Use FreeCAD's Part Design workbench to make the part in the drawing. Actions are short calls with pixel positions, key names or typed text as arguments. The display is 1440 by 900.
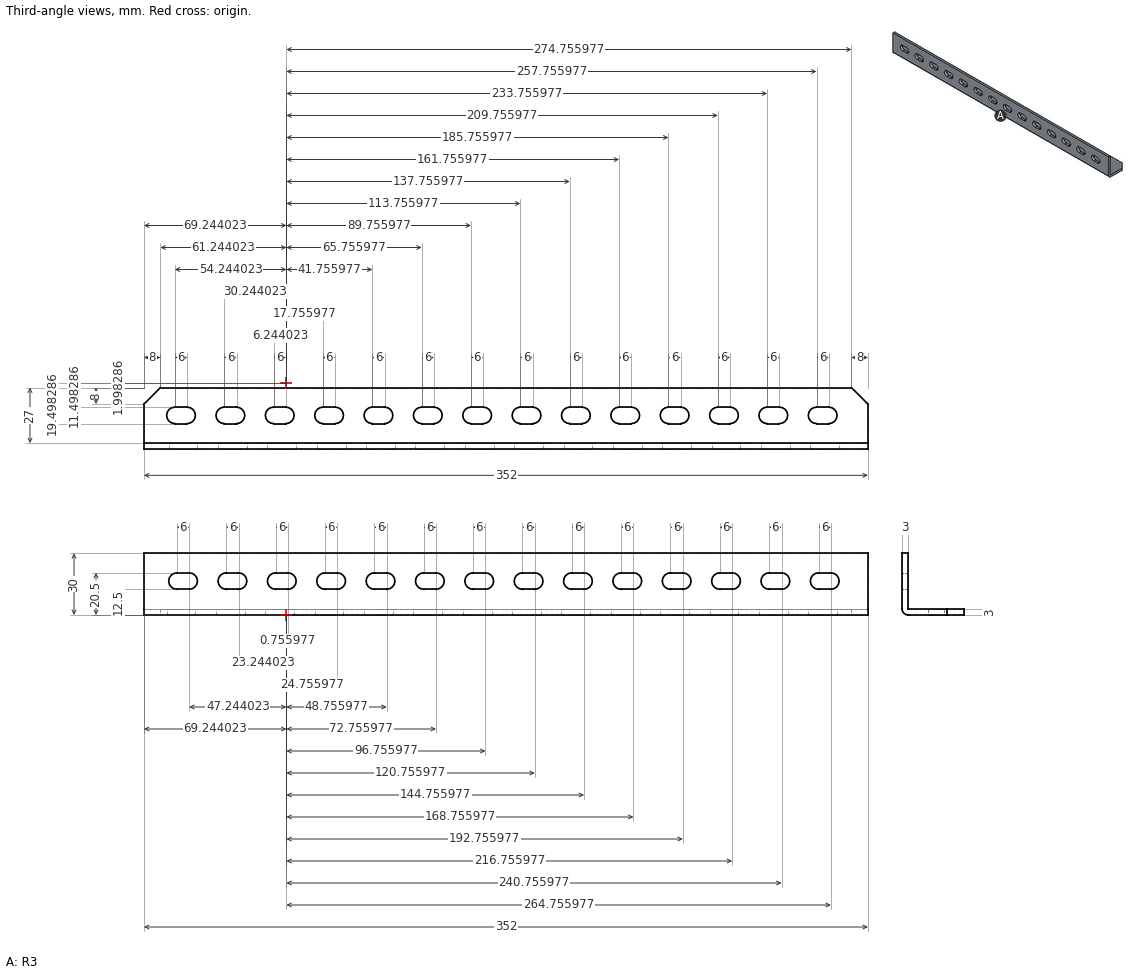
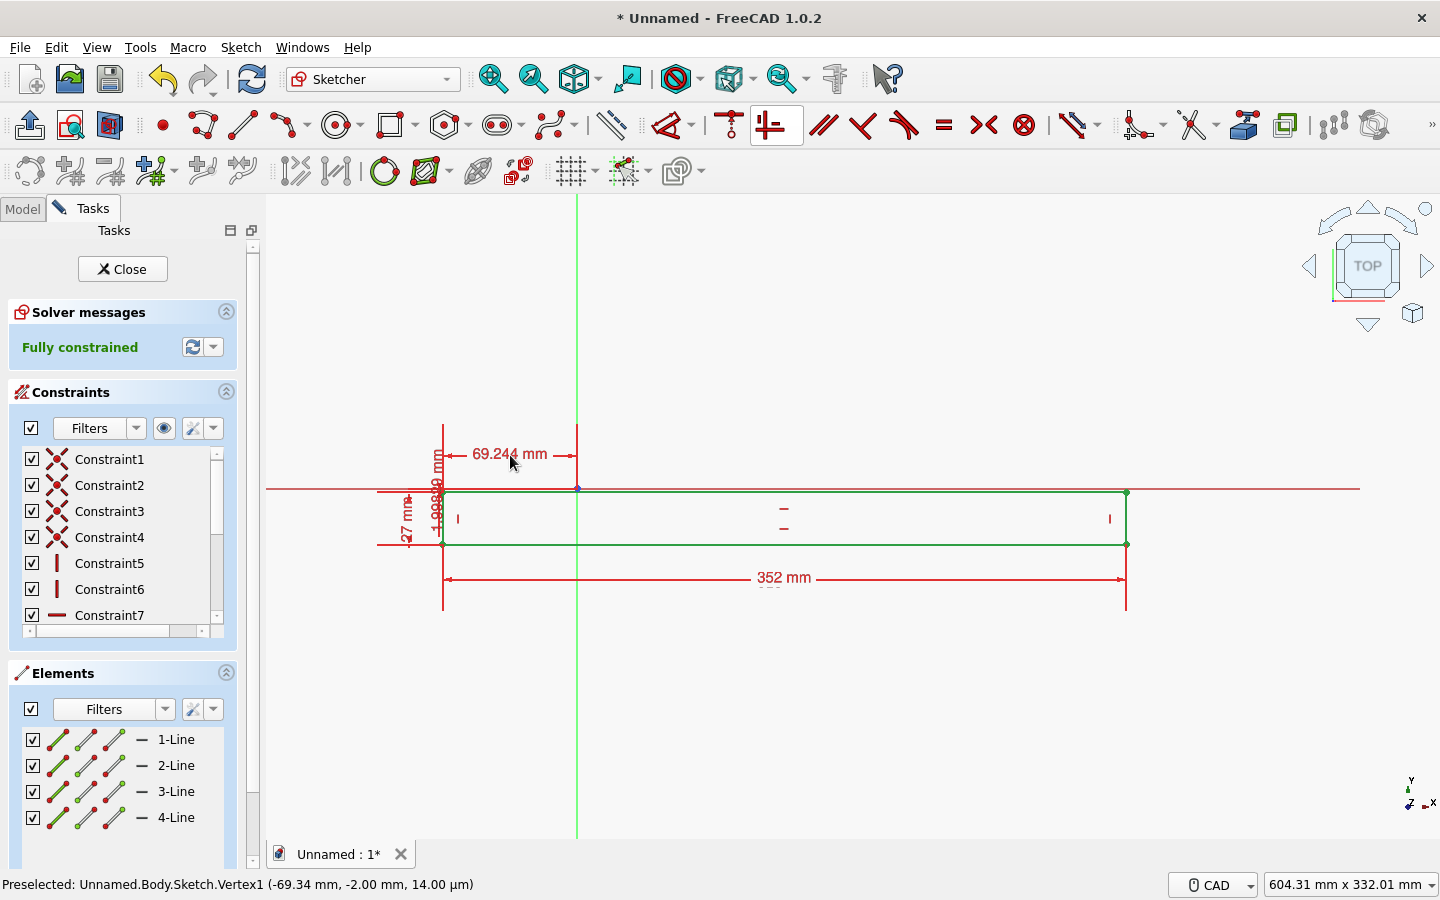
click(123, 269)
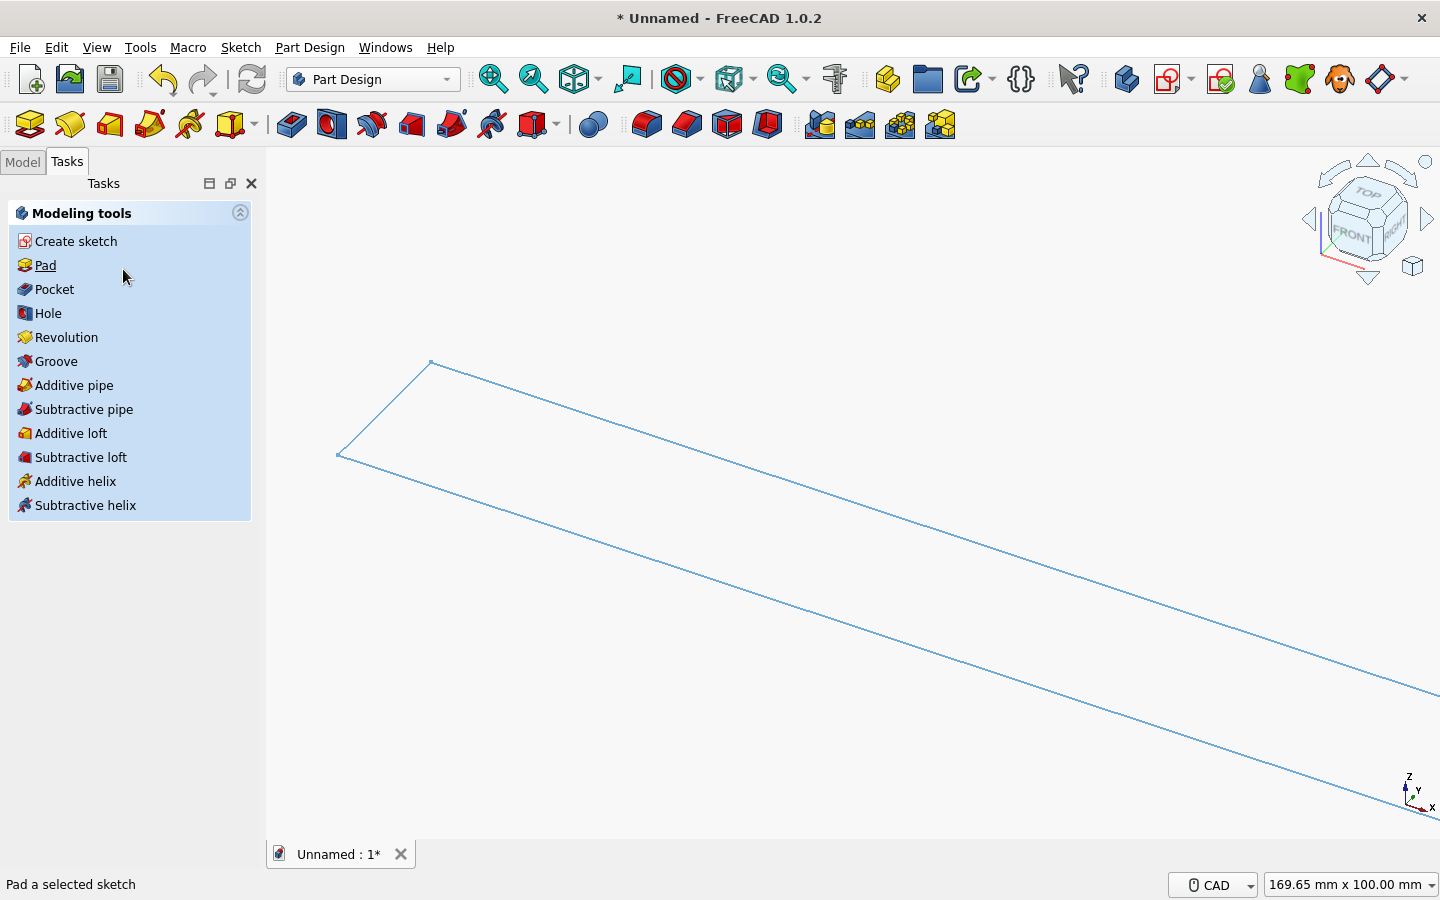
click(30, 124)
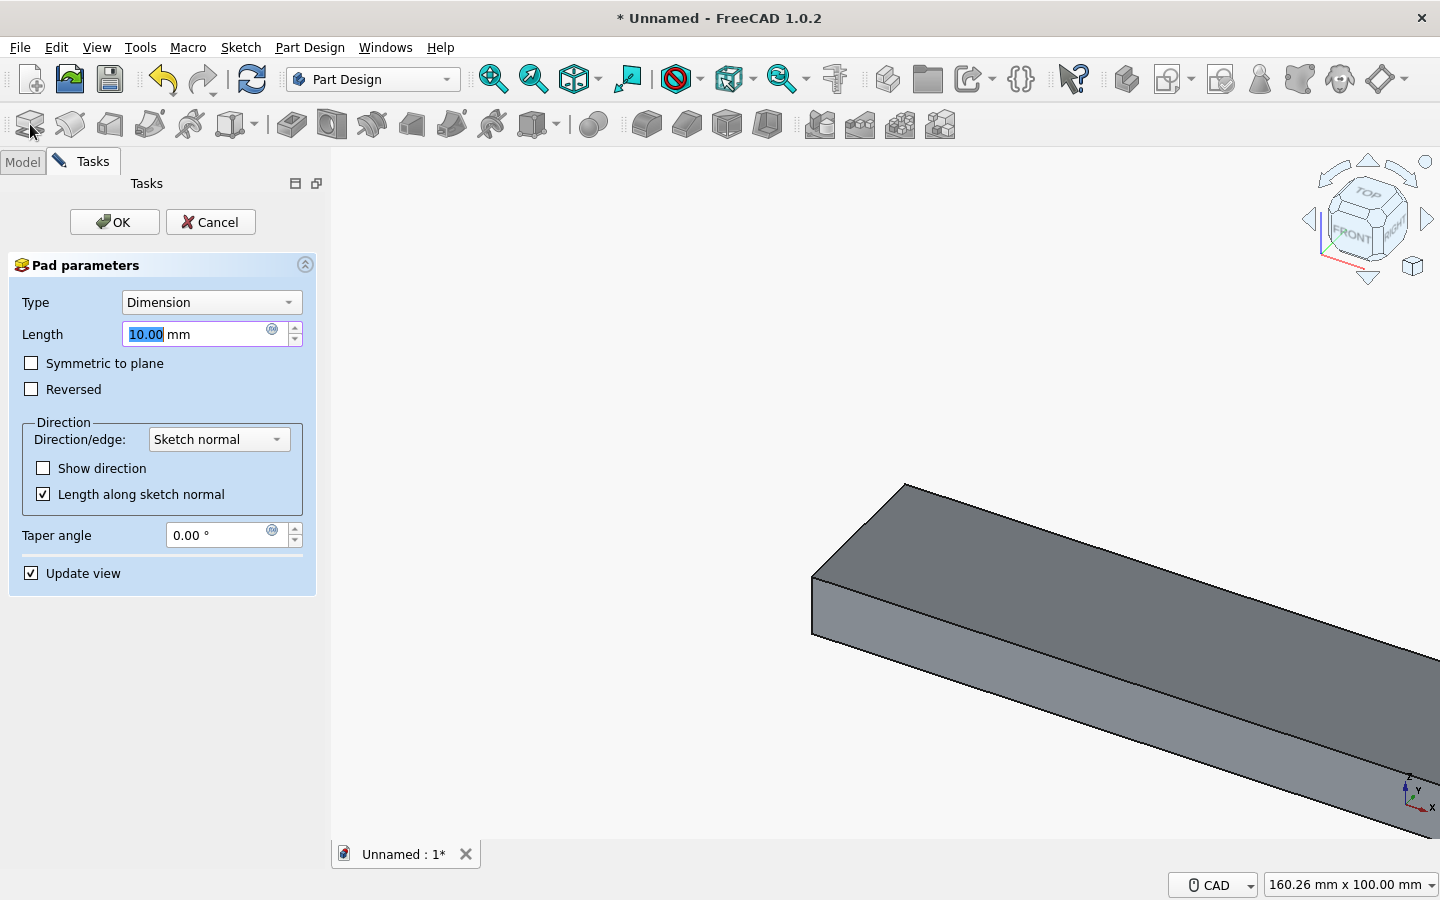
text(3)
key(Tab)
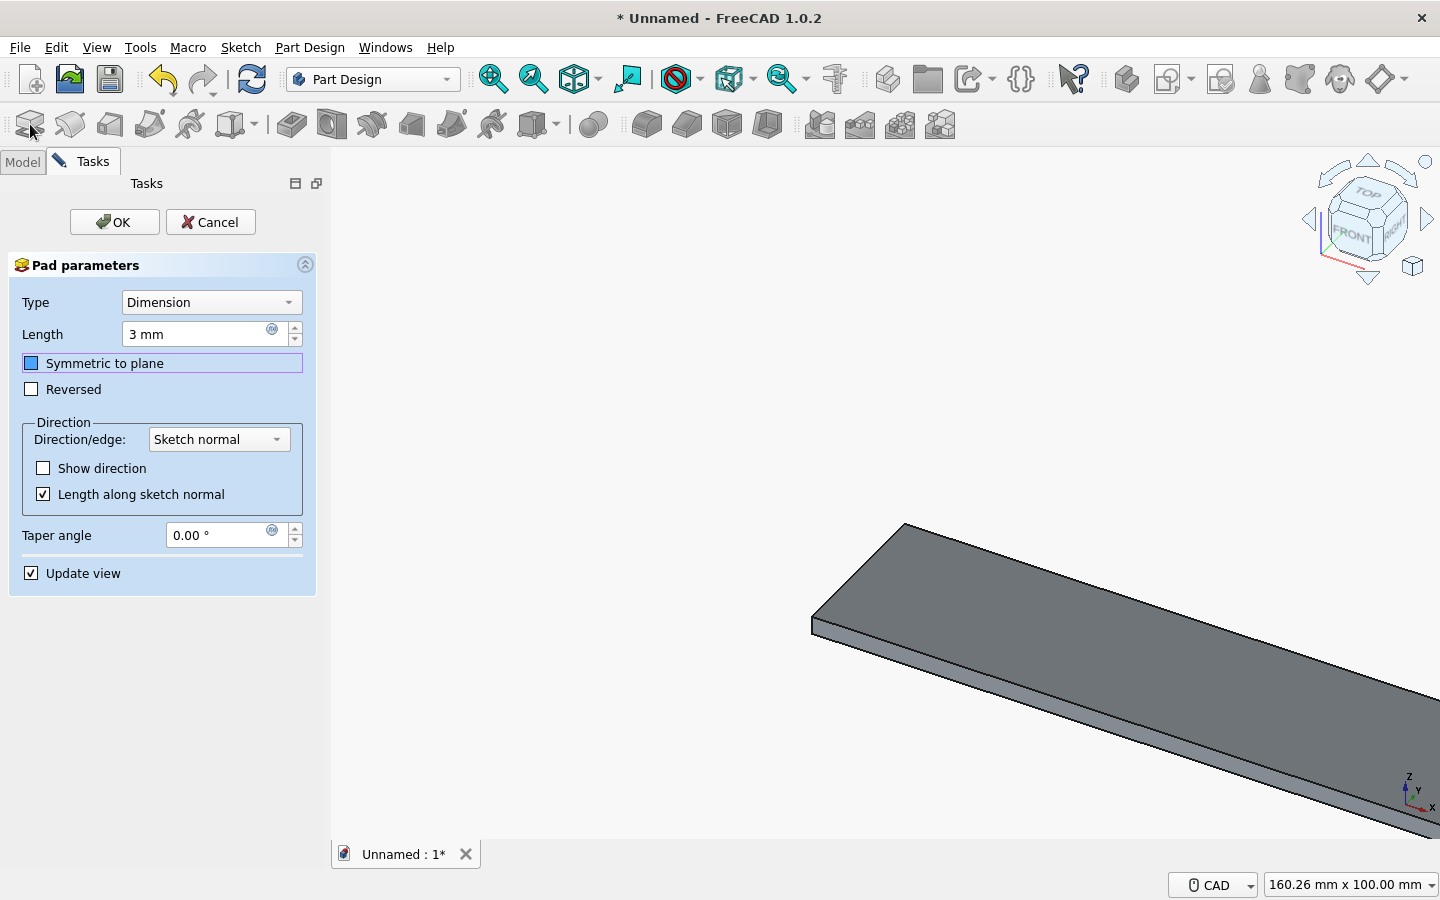
click(115, 222)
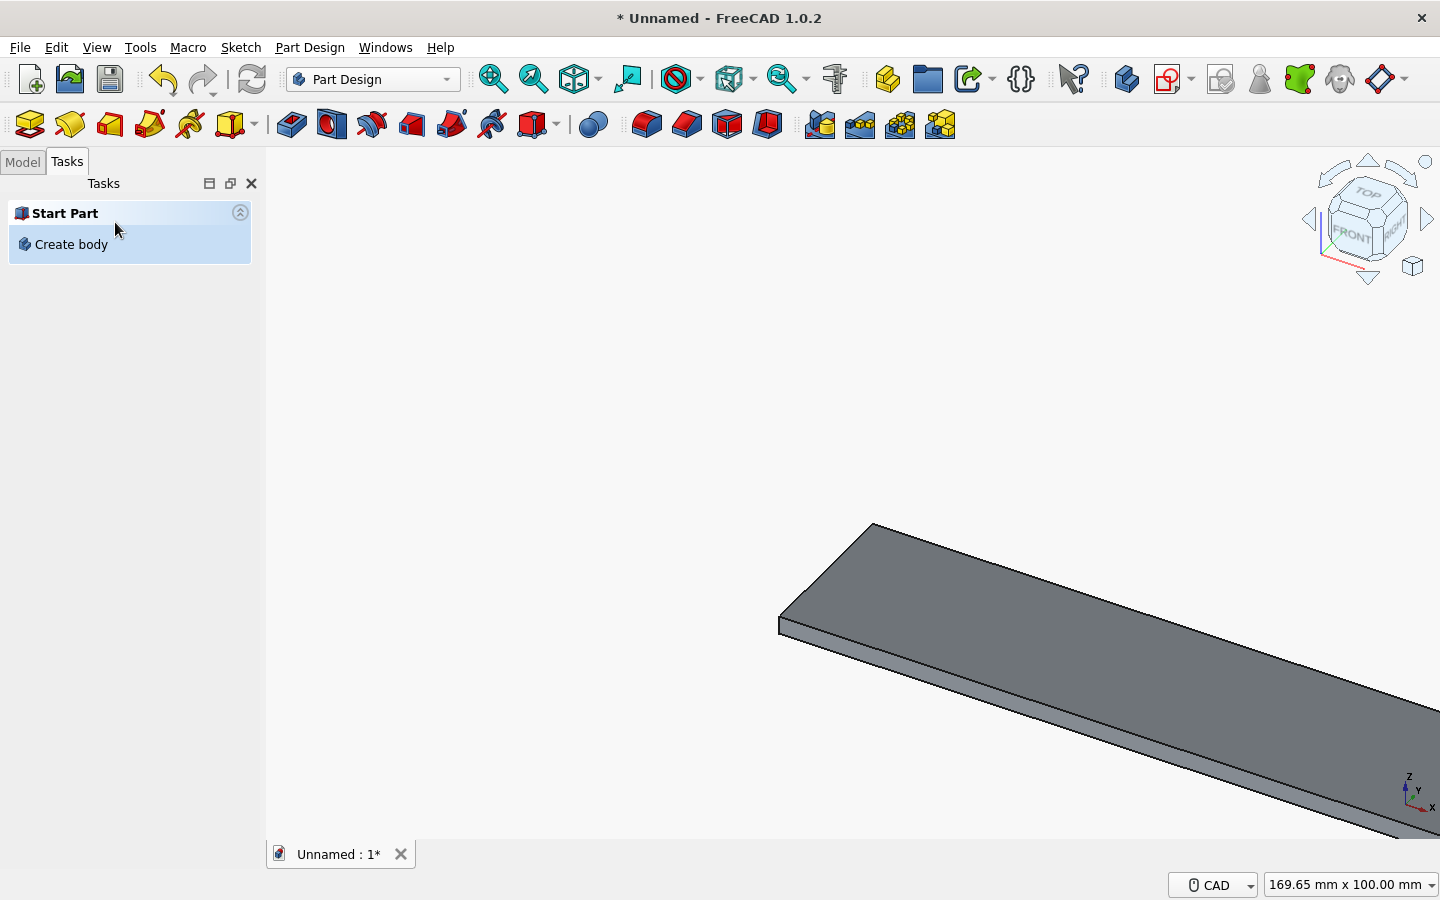
click(494, 80)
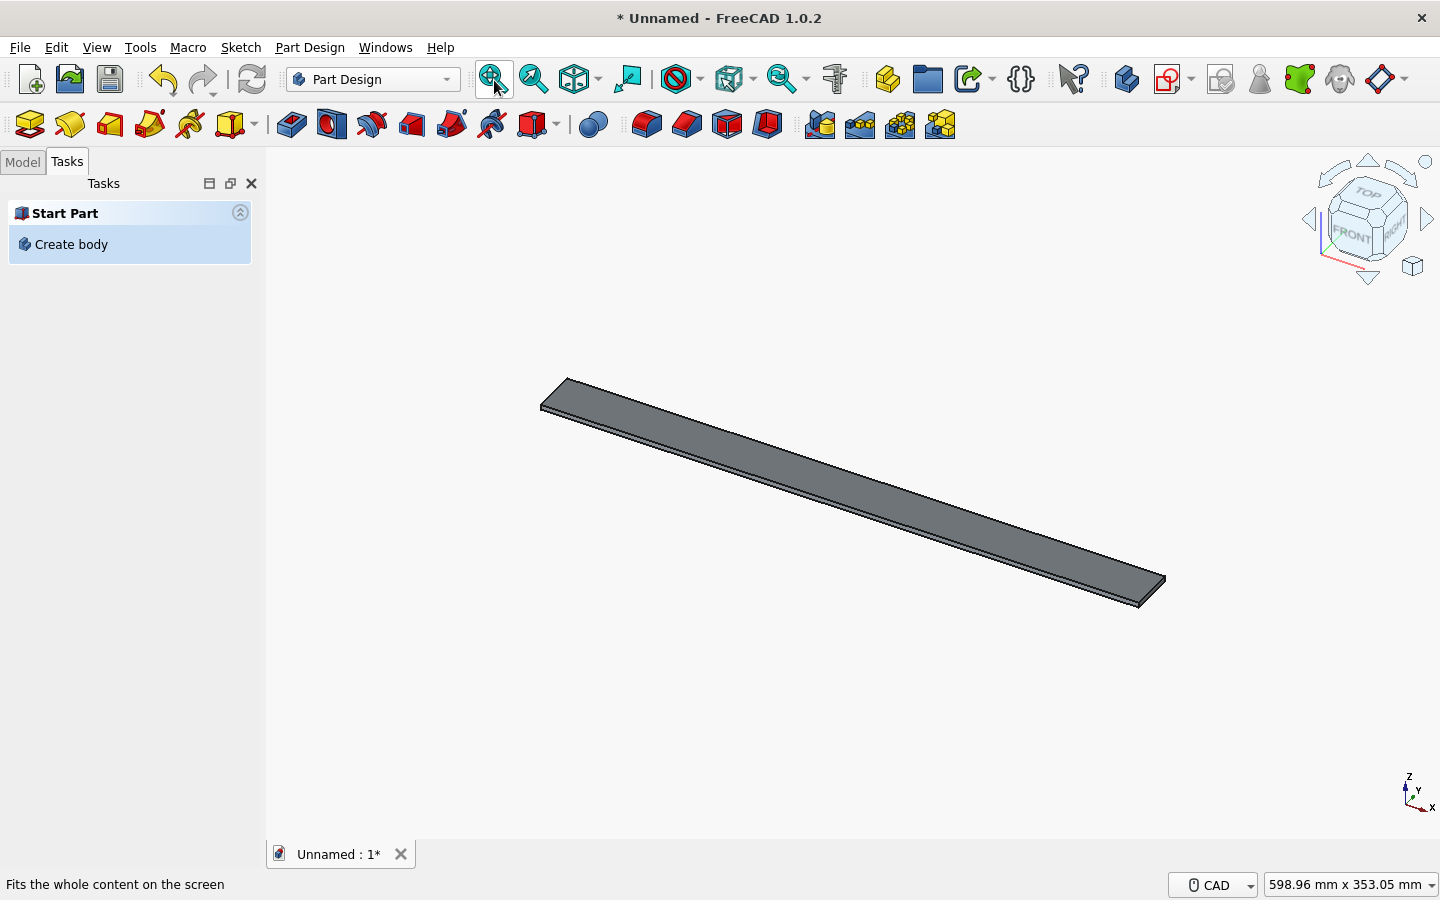
scroll(1096, 590, up, 8)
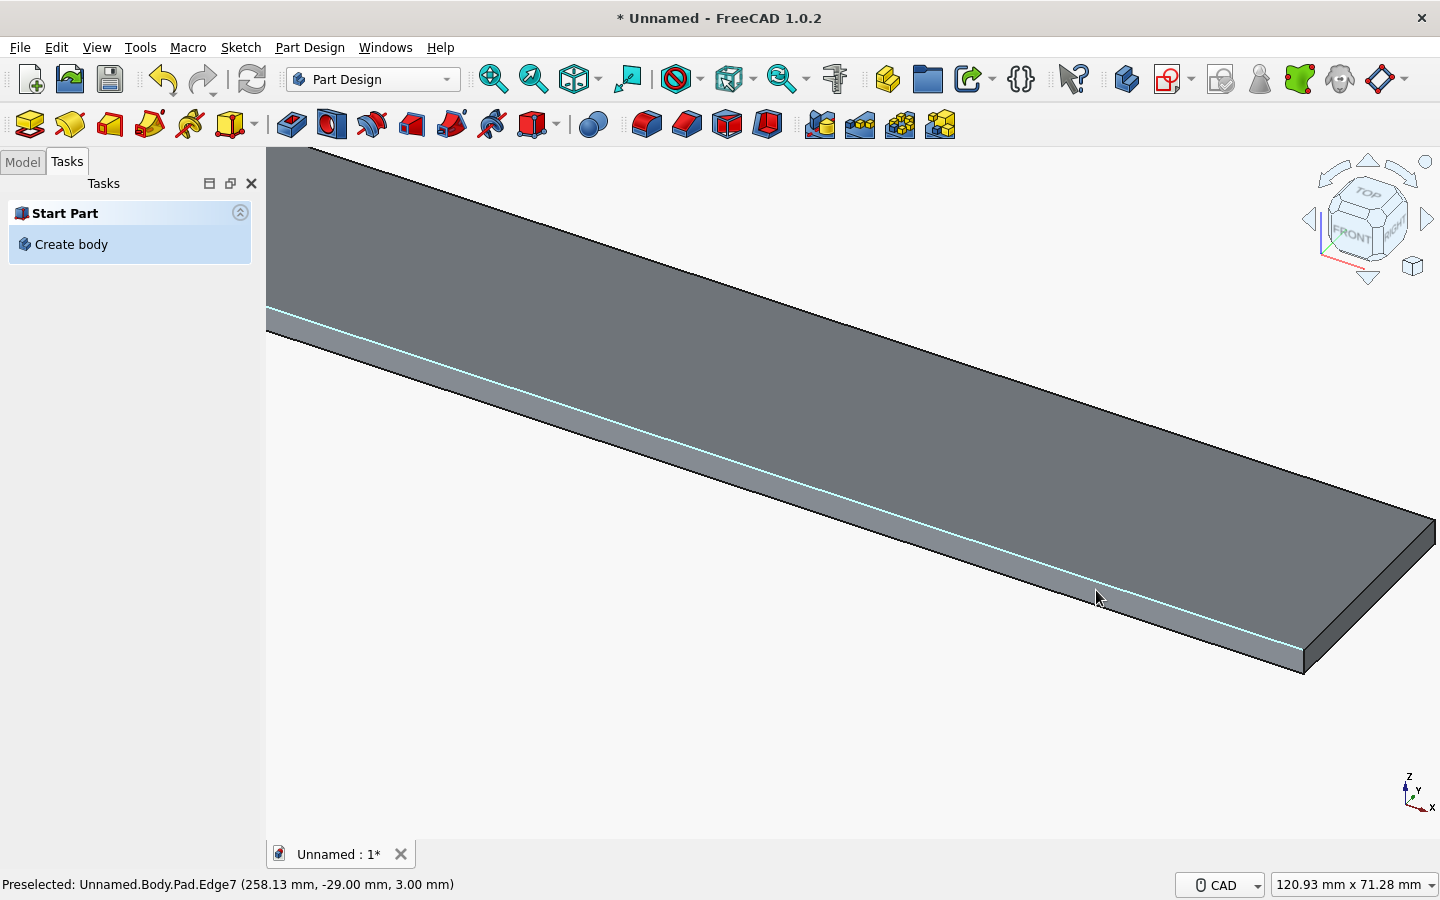
click(1092, 591)